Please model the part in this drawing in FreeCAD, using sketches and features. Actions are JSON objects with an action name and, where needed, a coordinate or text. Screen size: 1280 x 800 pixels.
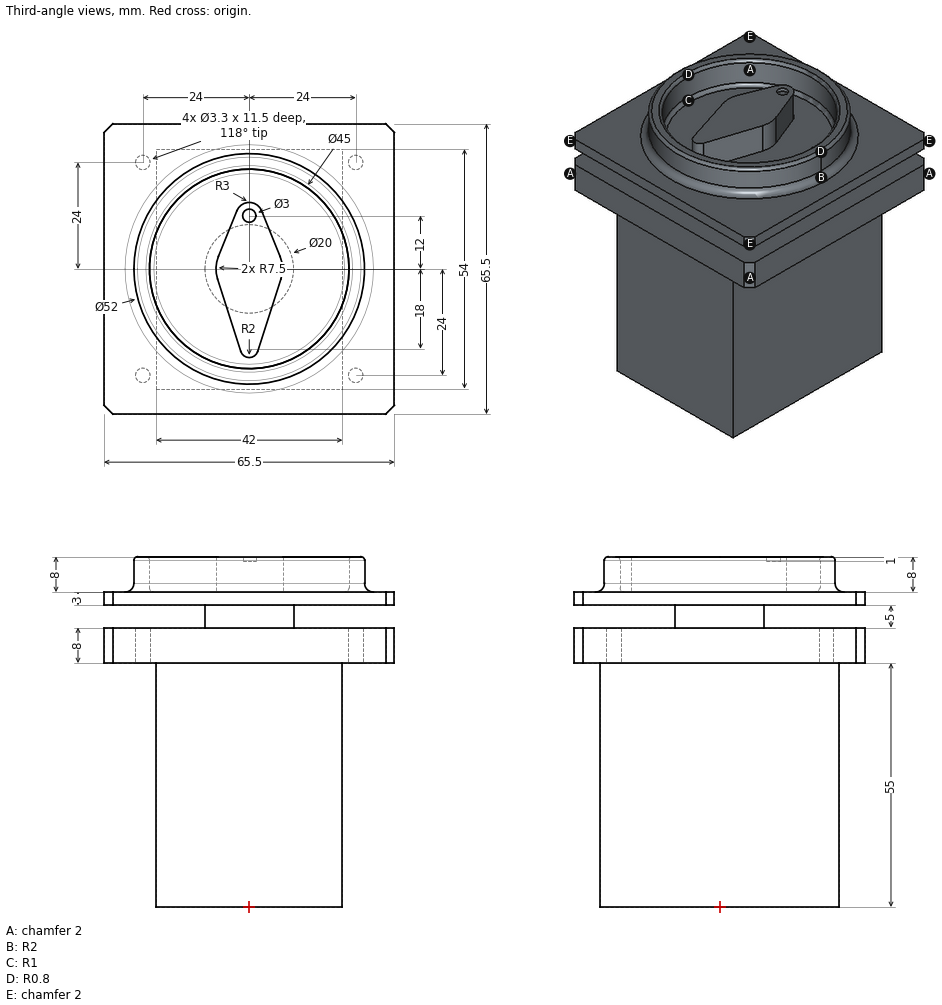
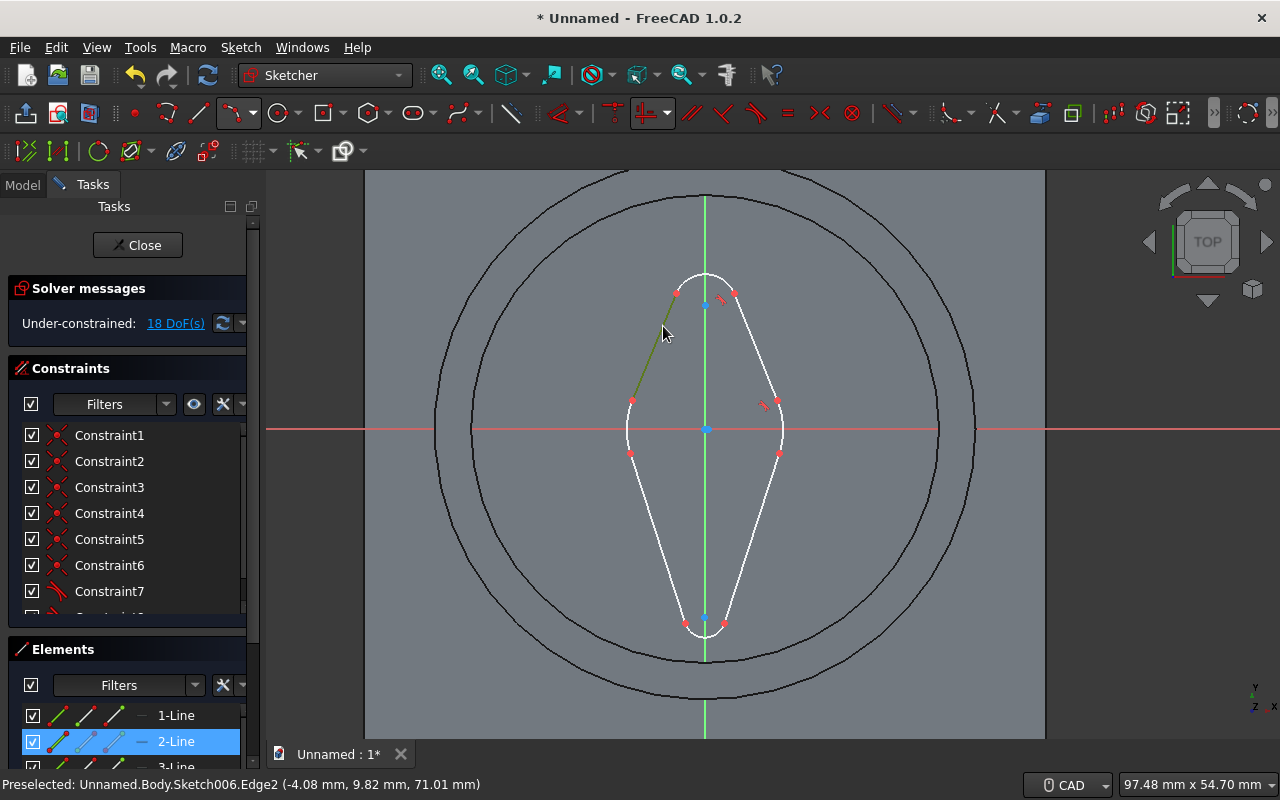
{"action": "left_click", "coordinate": [720, 278]}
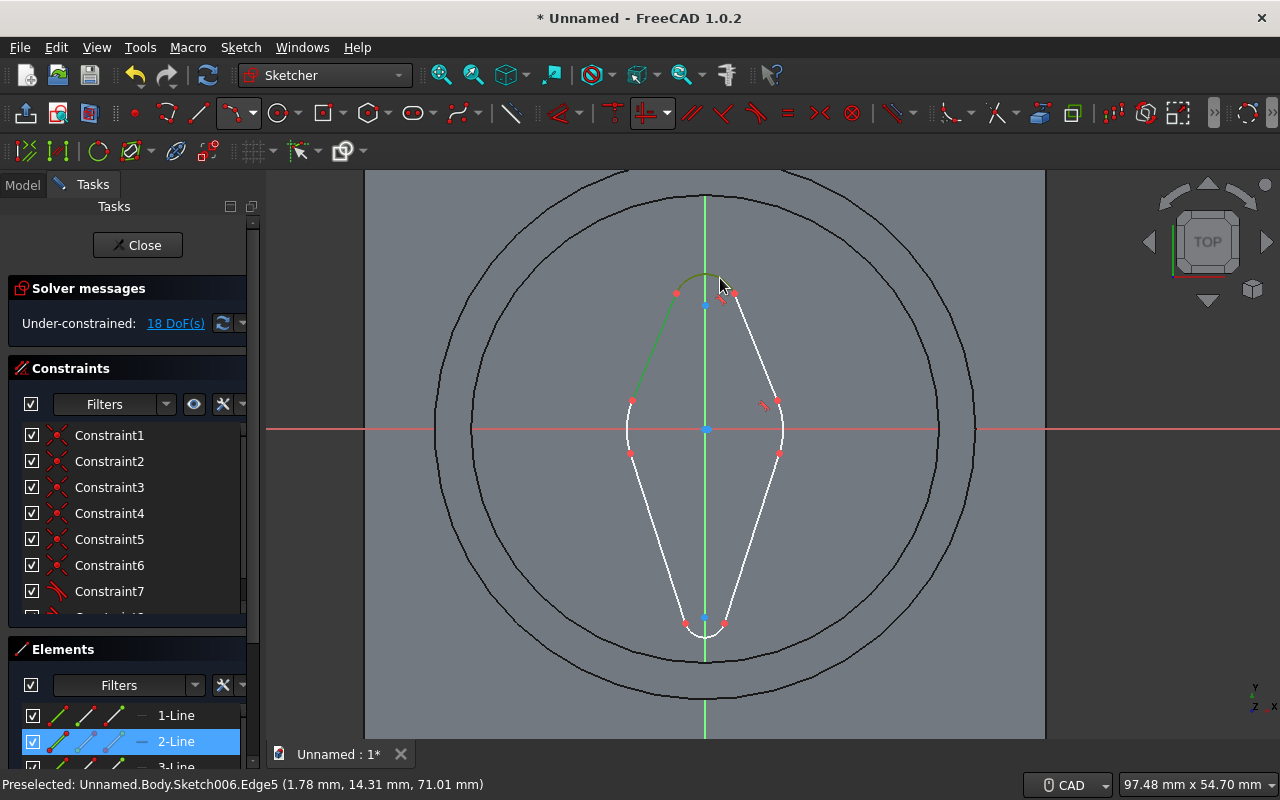
{"action": "left_click", "coordinate": [756, 114]}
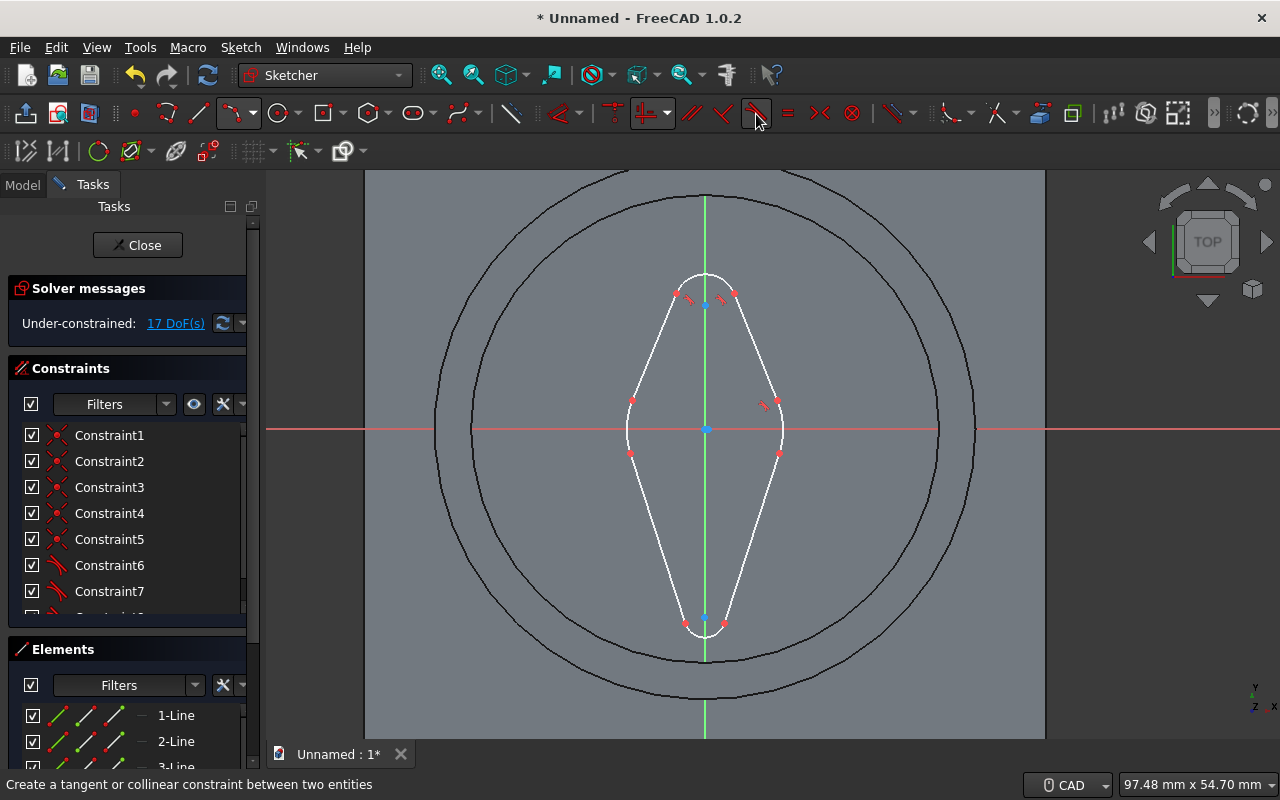
{"action": "left_click", "coordinate": [663, 326]}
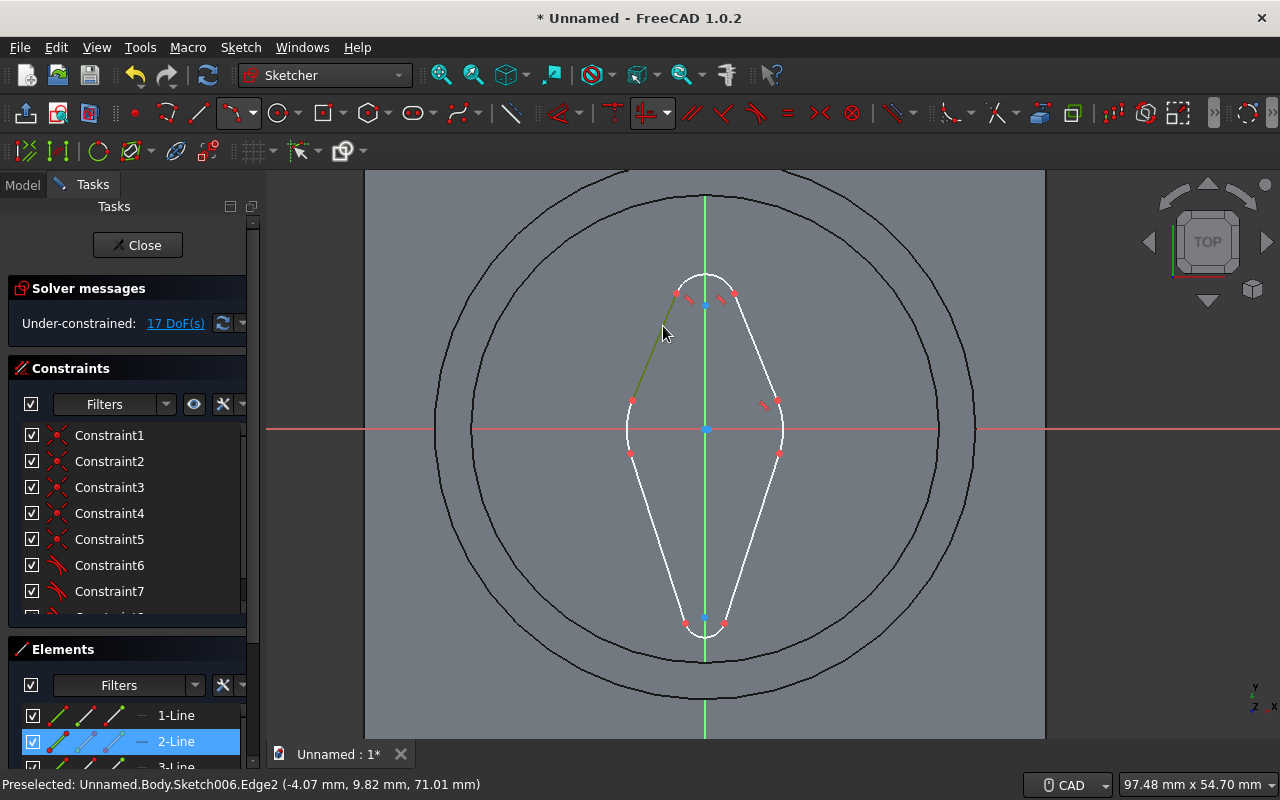
{"action": "left_click", "coordinate": [628, 416]}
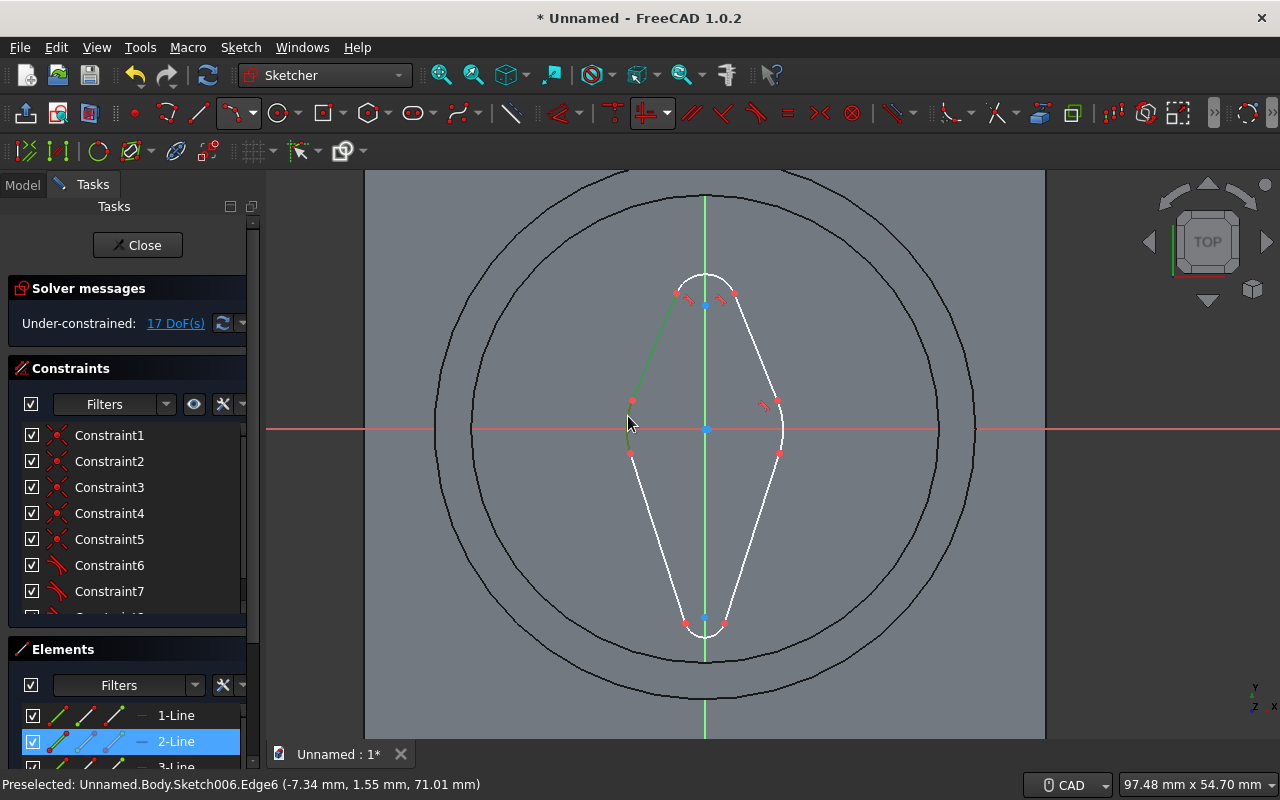
{"action": "left_click", "coordinate": [756, 114]}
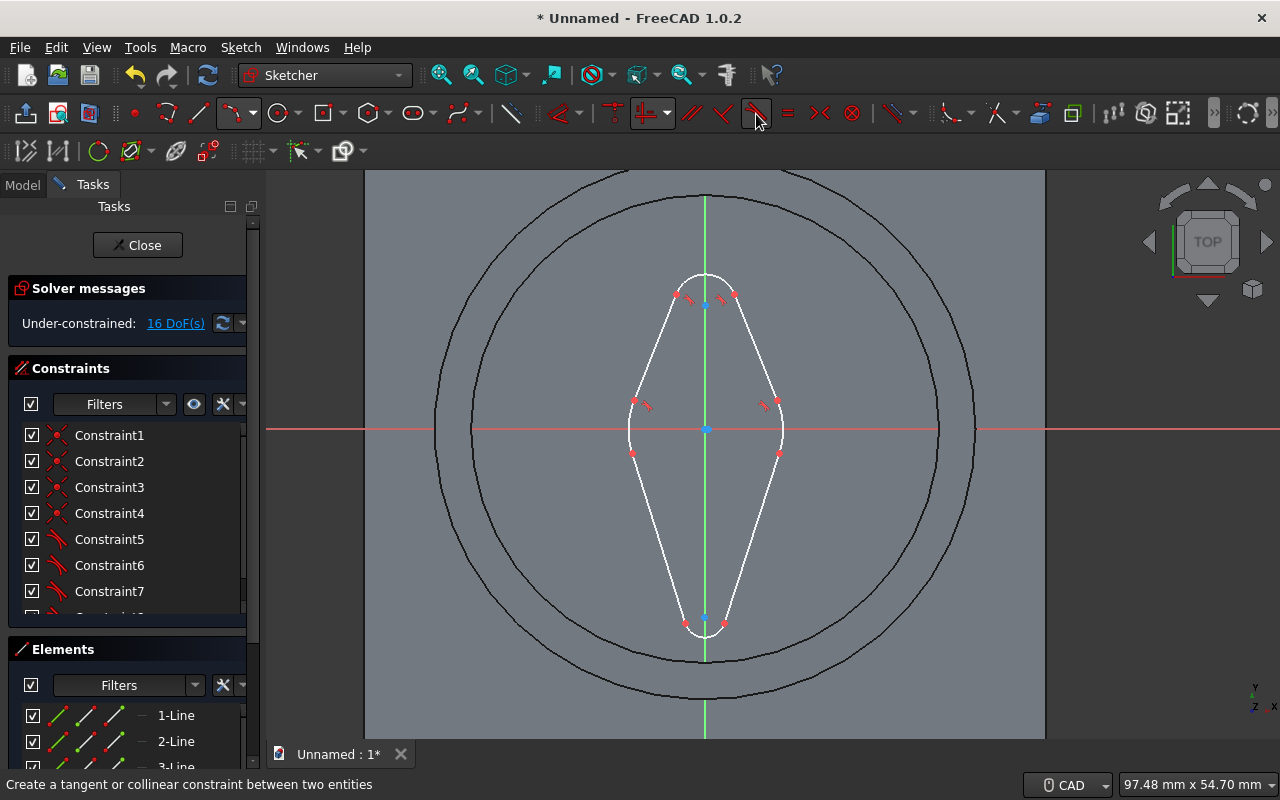
{"action": "left_click", "coordinate": [648, 505]}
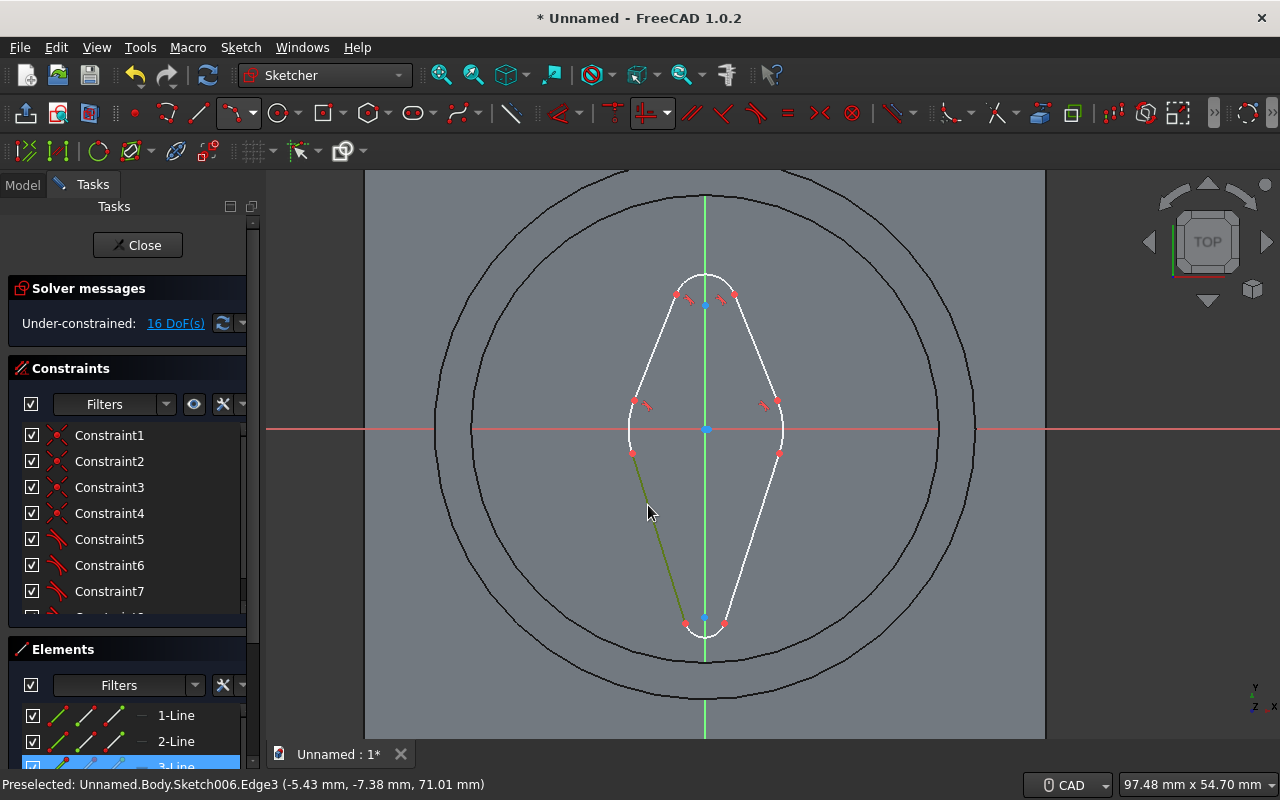
{"action": "left_click", "coordinate": [630, 416]}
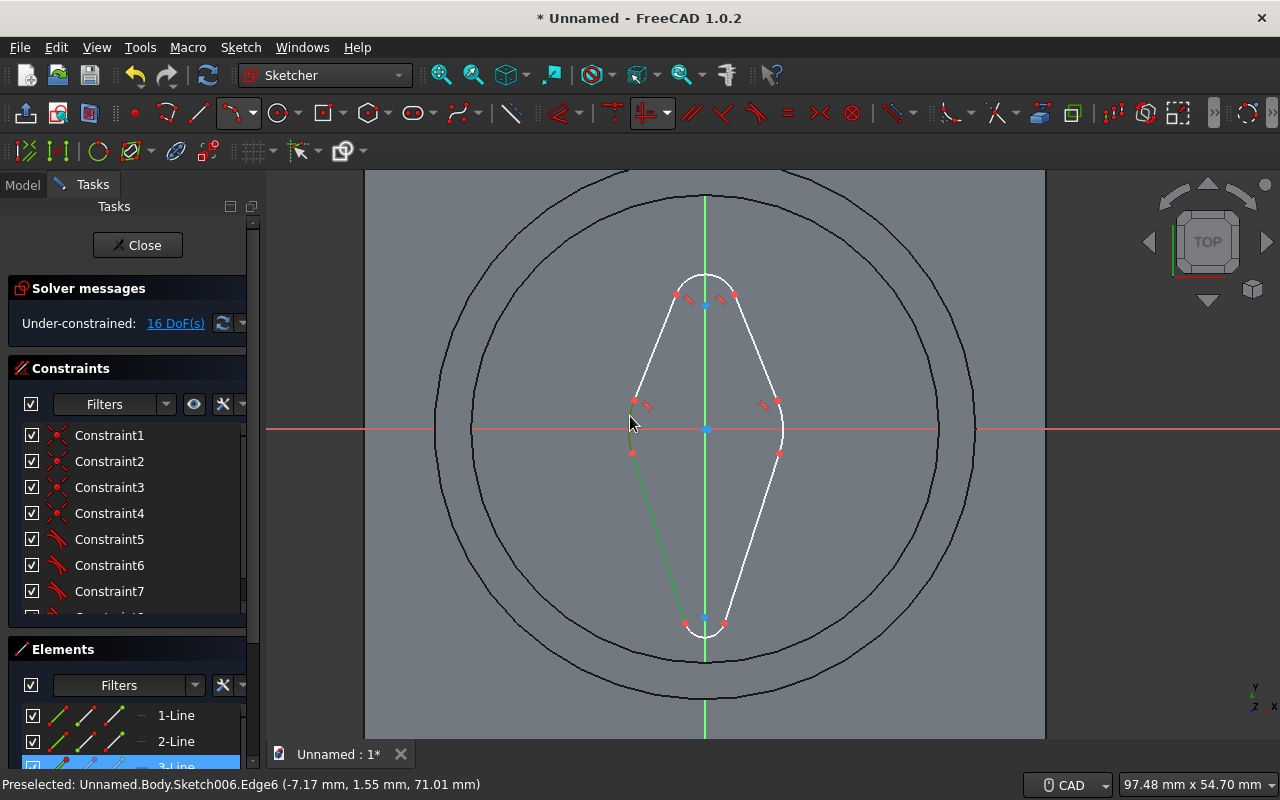
{"action": "left_click", "coordinate": [756, 114]}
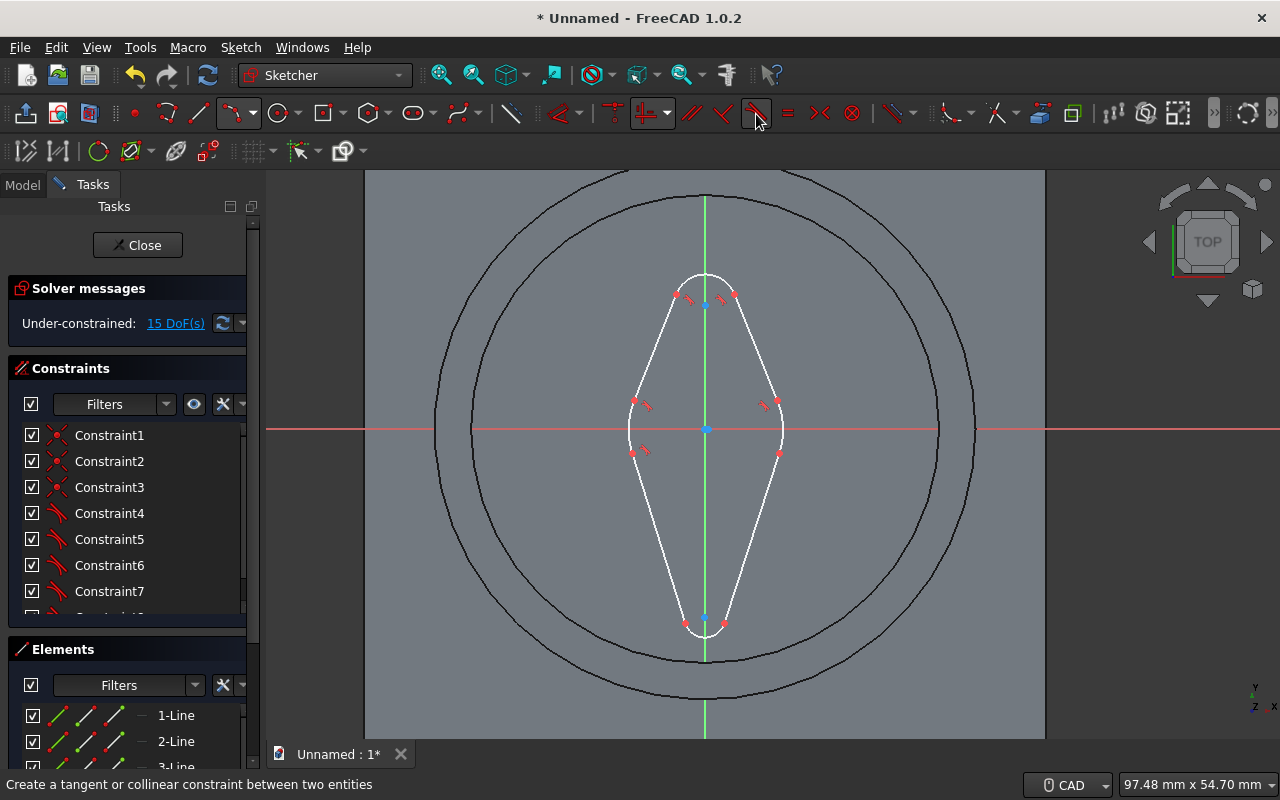
{"action": "left_click", "coordinate": [648, 505]}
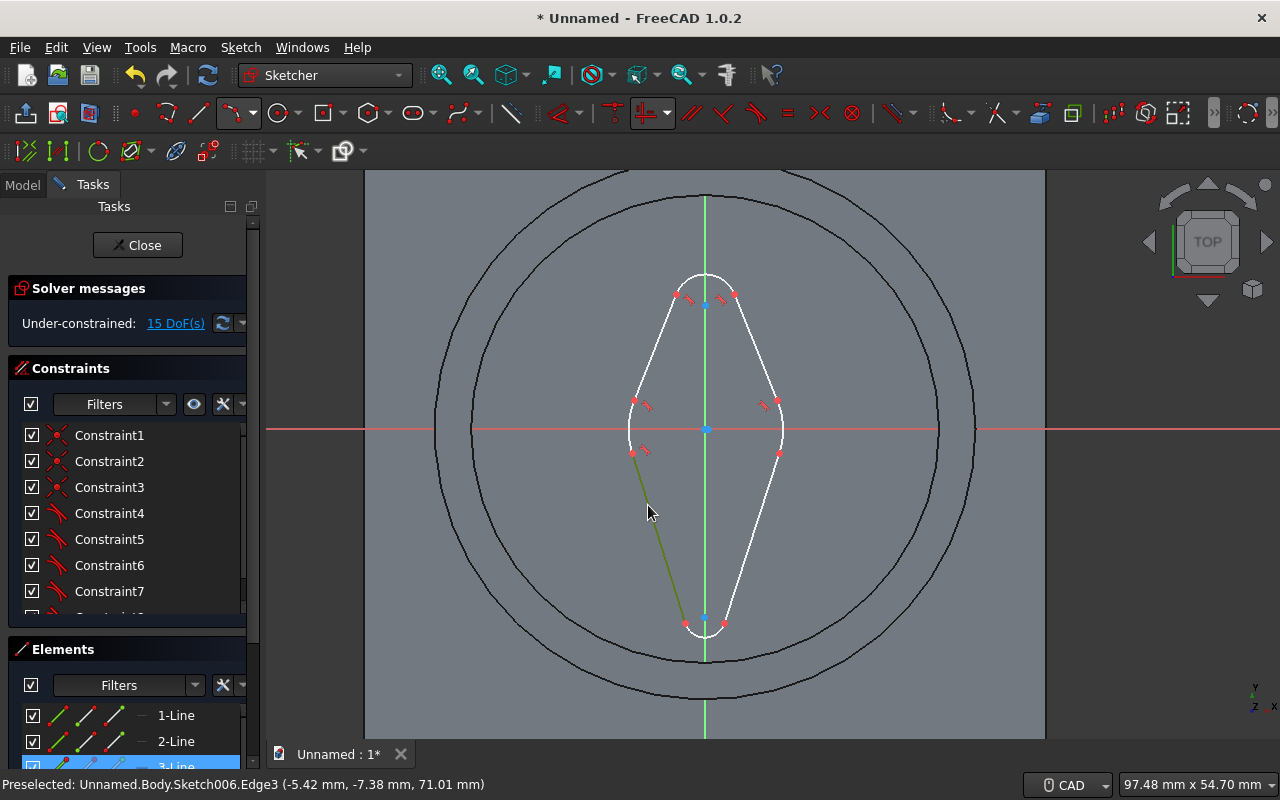
{"action": "scroll", "coordinate": [695, 635], "scroll_direction": "up", "scroll_amount": 2}